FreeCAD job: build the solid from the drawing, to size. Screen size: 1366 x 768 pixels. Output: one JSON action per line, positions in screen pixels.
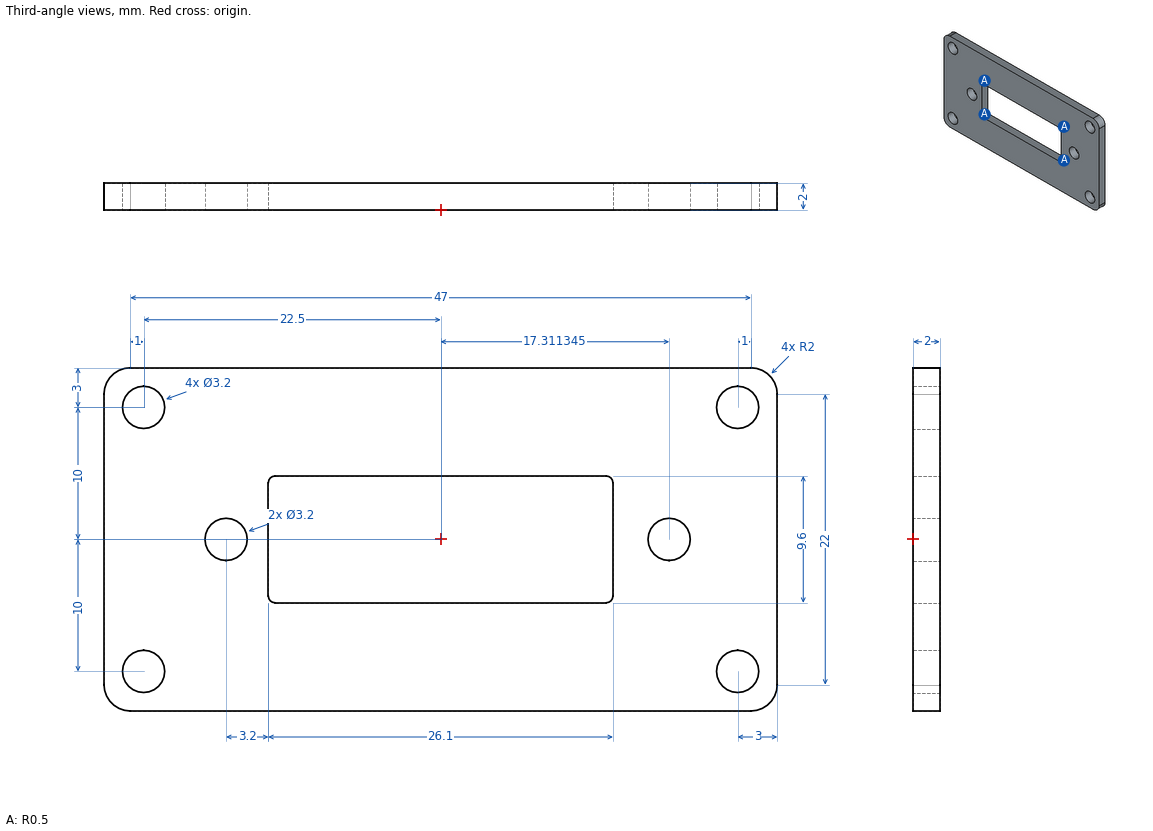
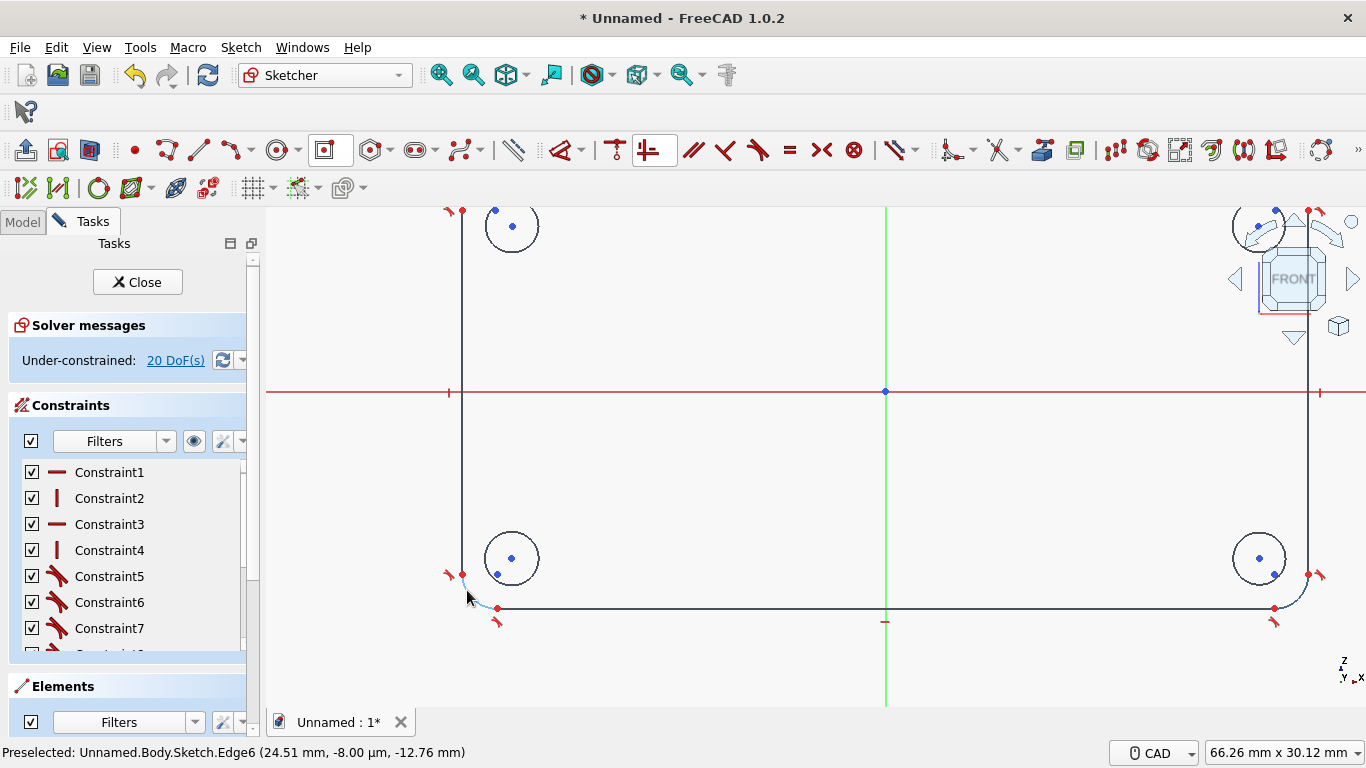
{"action": "left_click", "coordinate": [466, 590]}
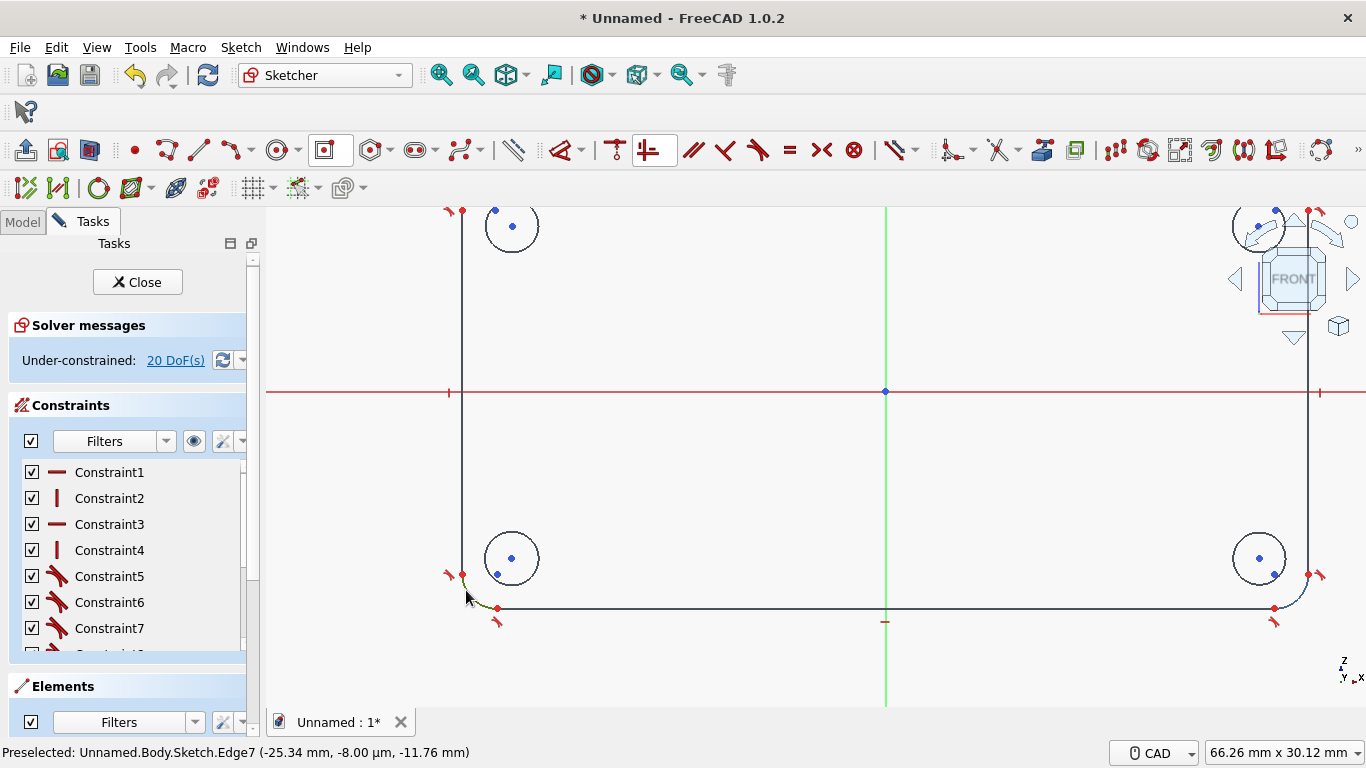
{"action": "scroll", "coordinate": [467, 590], "scroll_direction": "down", "scroll_amount": 2}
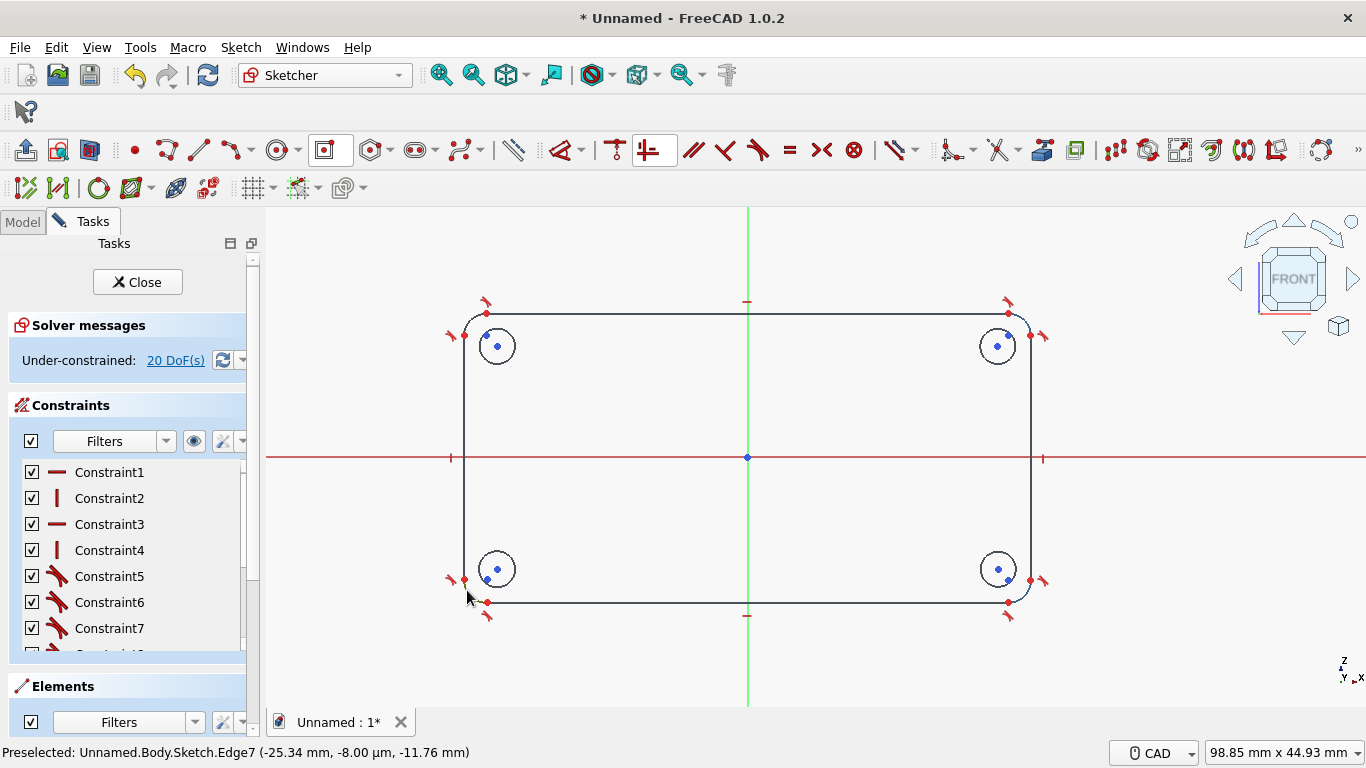
{"action": "scroll", "coordinate": [476, 316], "scroll_direction": "up", "scroll_amount": 2}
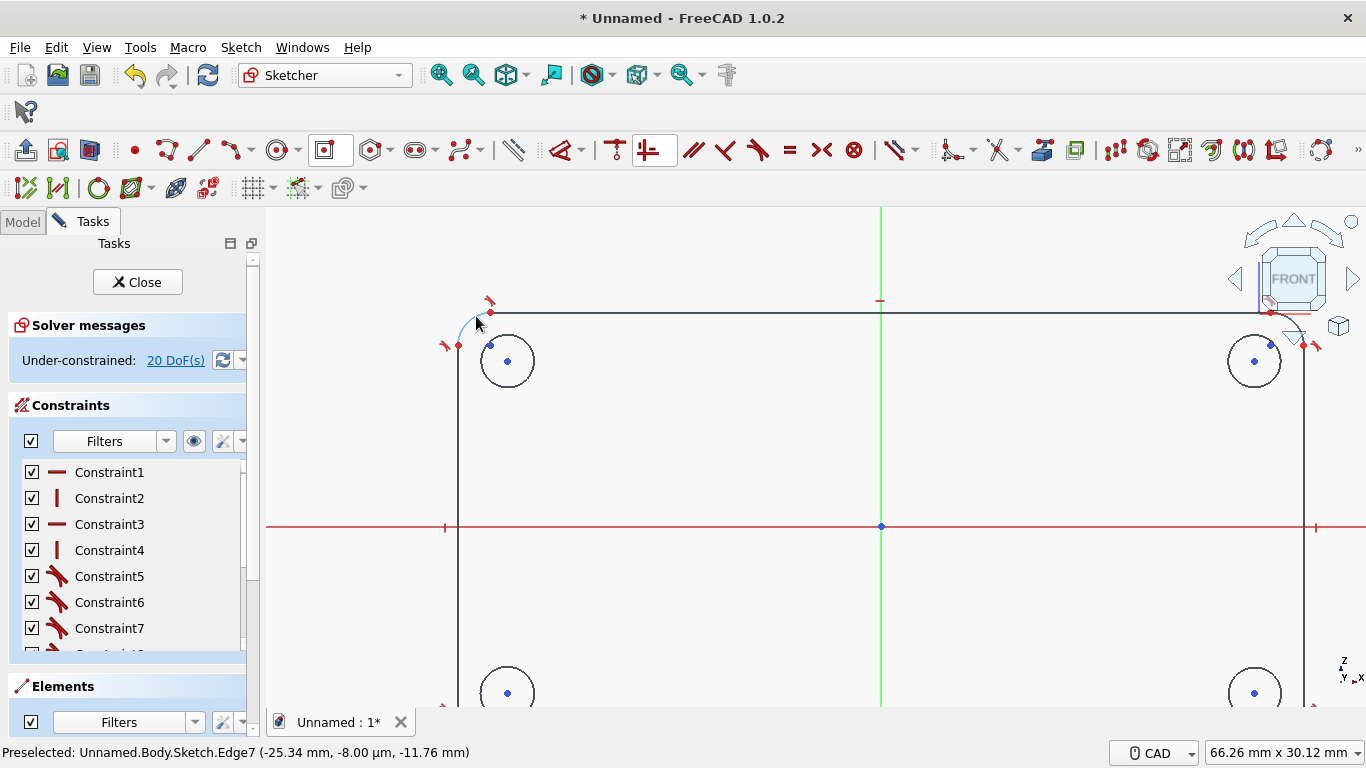
{"action": "left_click", "coordinate": [476, 316]}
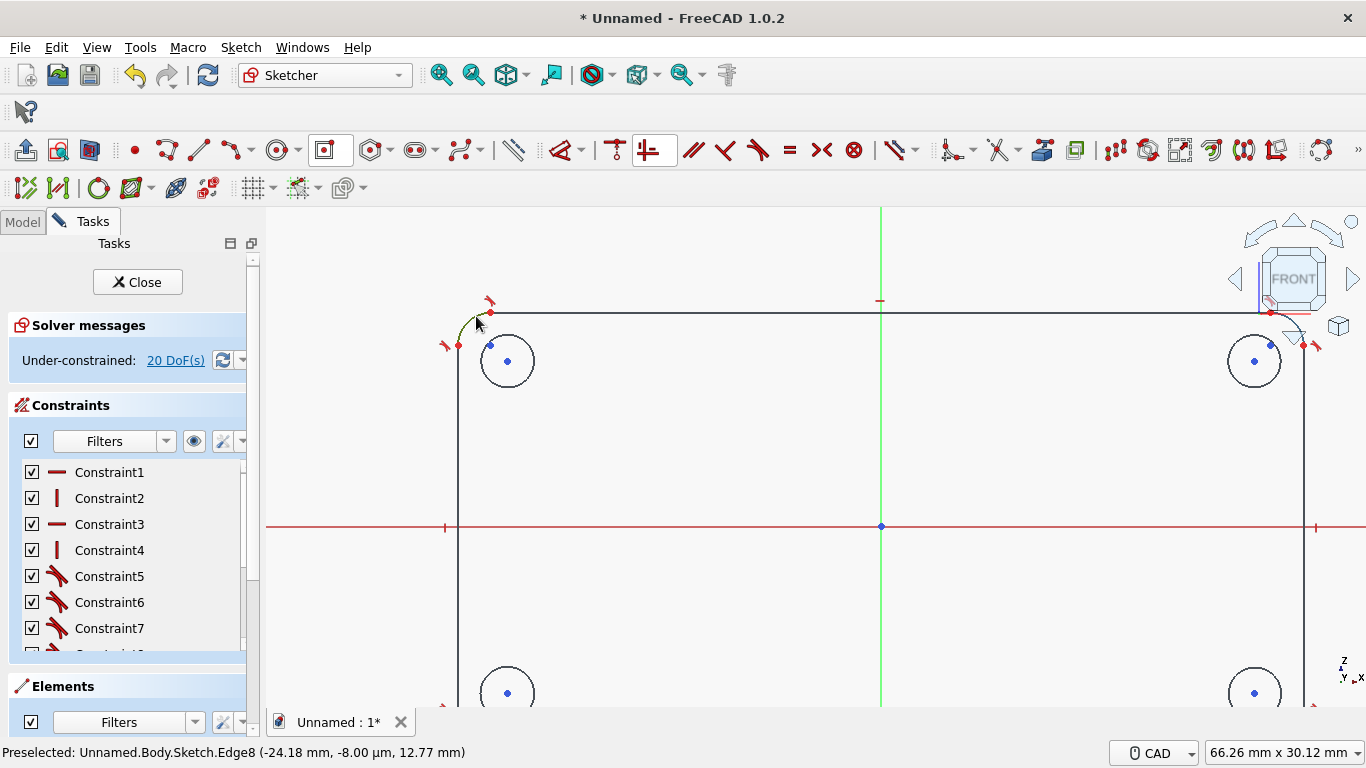
{"action": "left_click", "coordinate": [790, 150]}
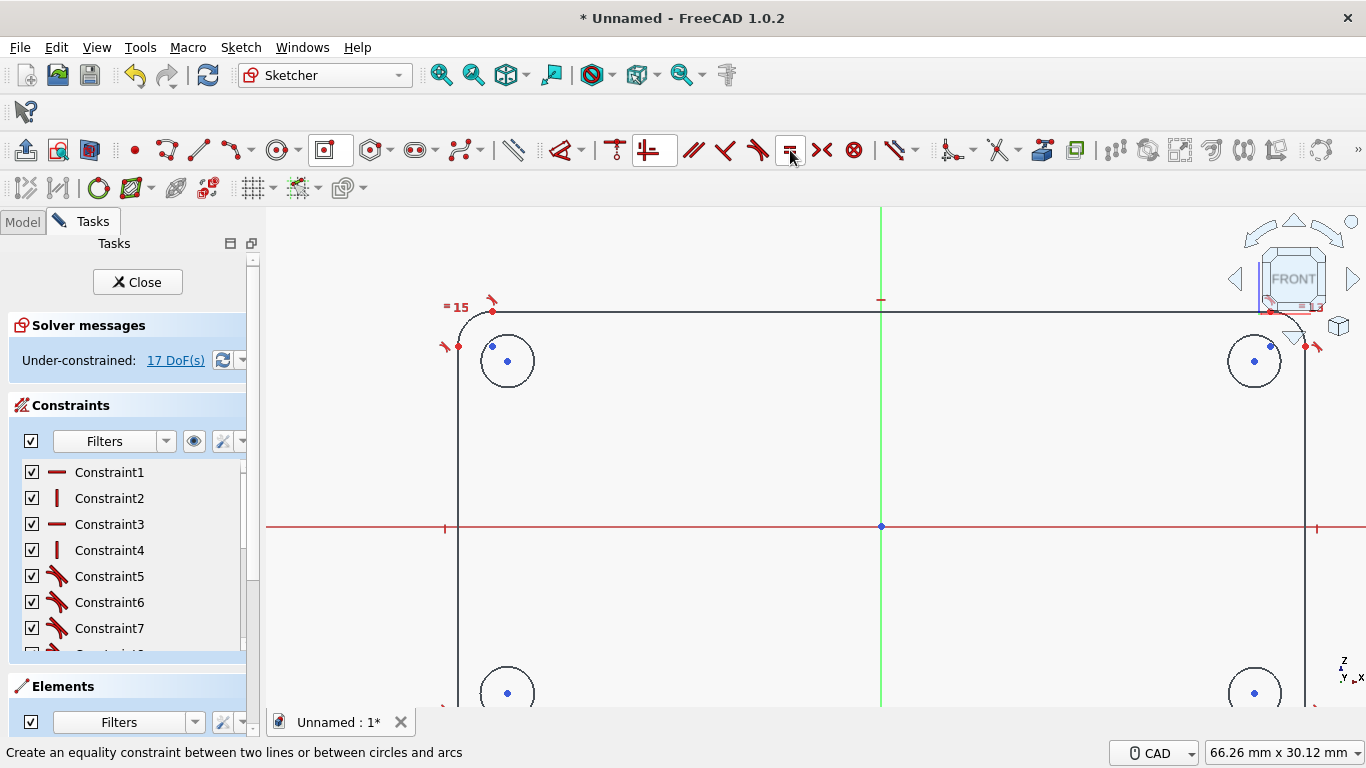
{"action": "left_click", "coordinate": [526, 342]}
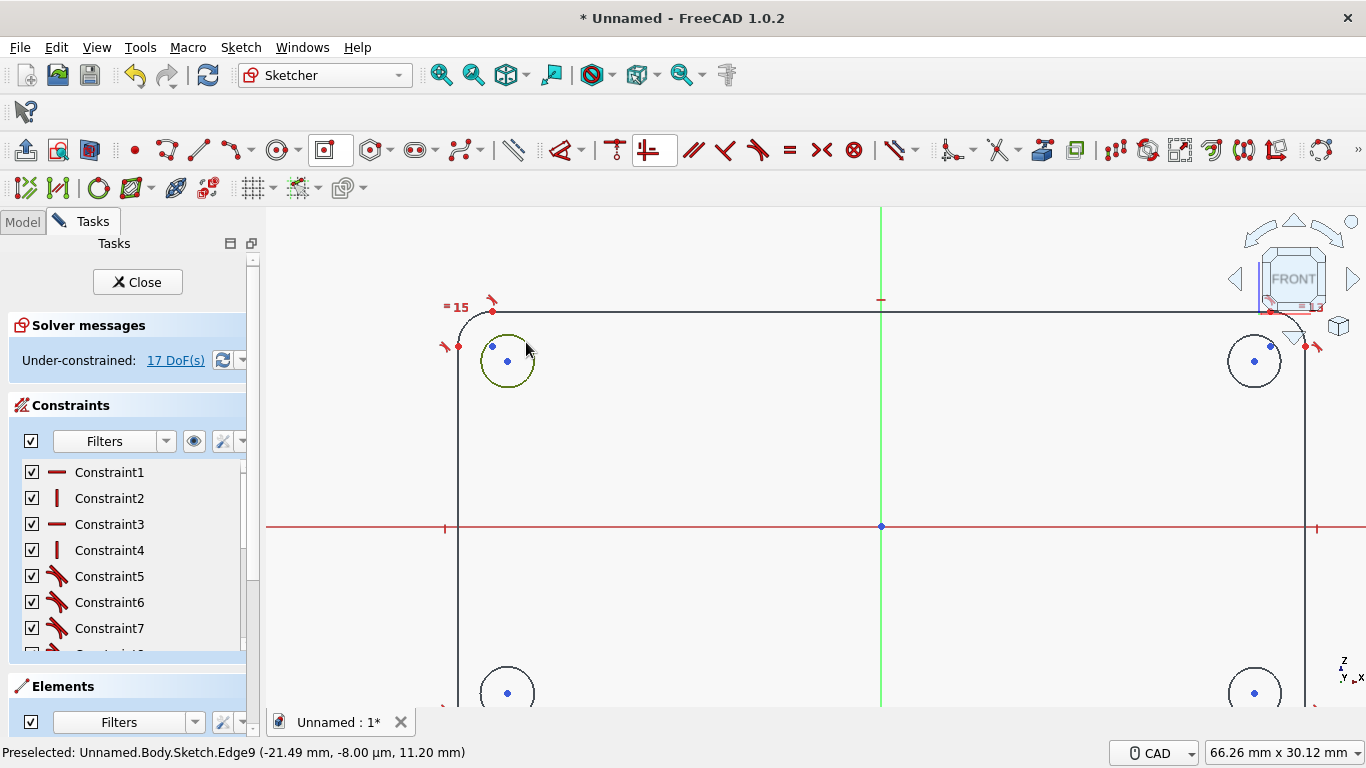
{"action": "scroll", "coordinate": [476, 315], "scroll_direction": "down", "scroll_amount": 2}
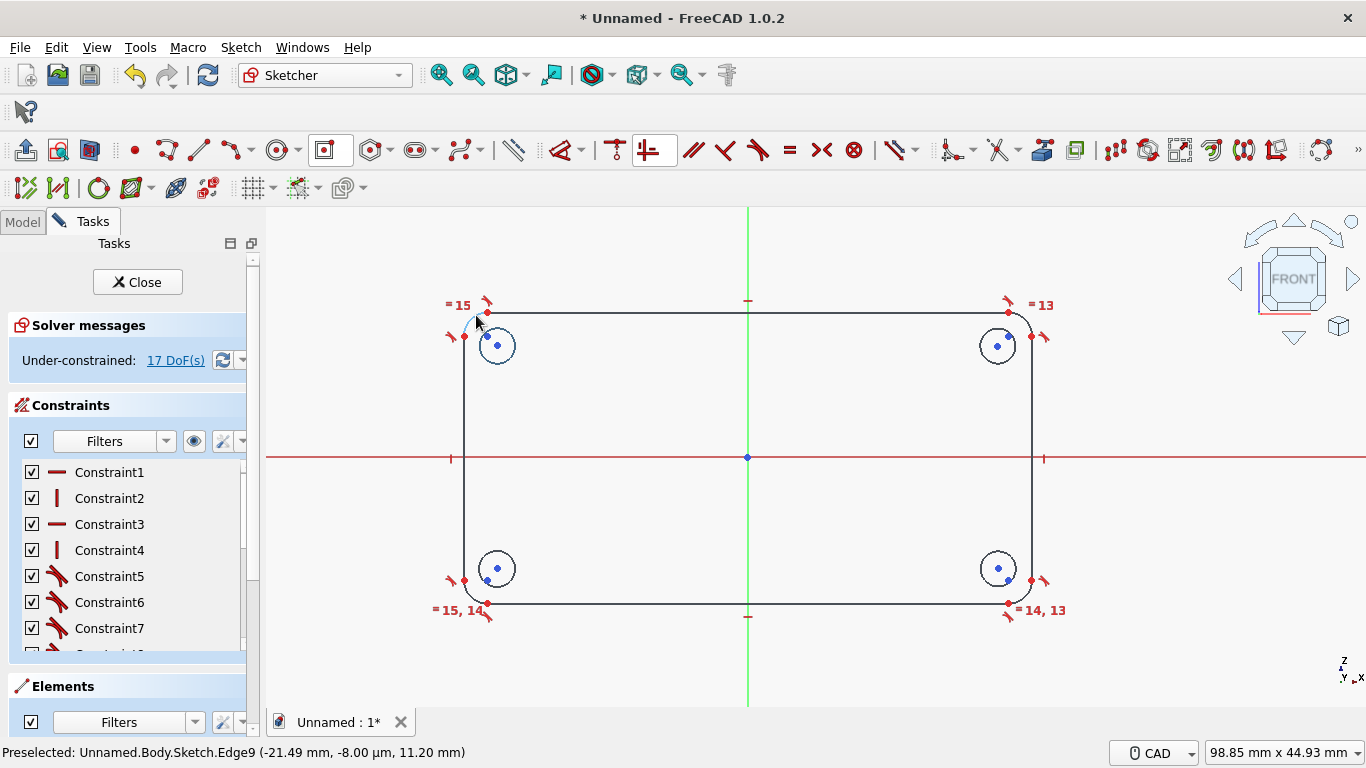
{"action": "left_click", "coordinate": [985, 334]}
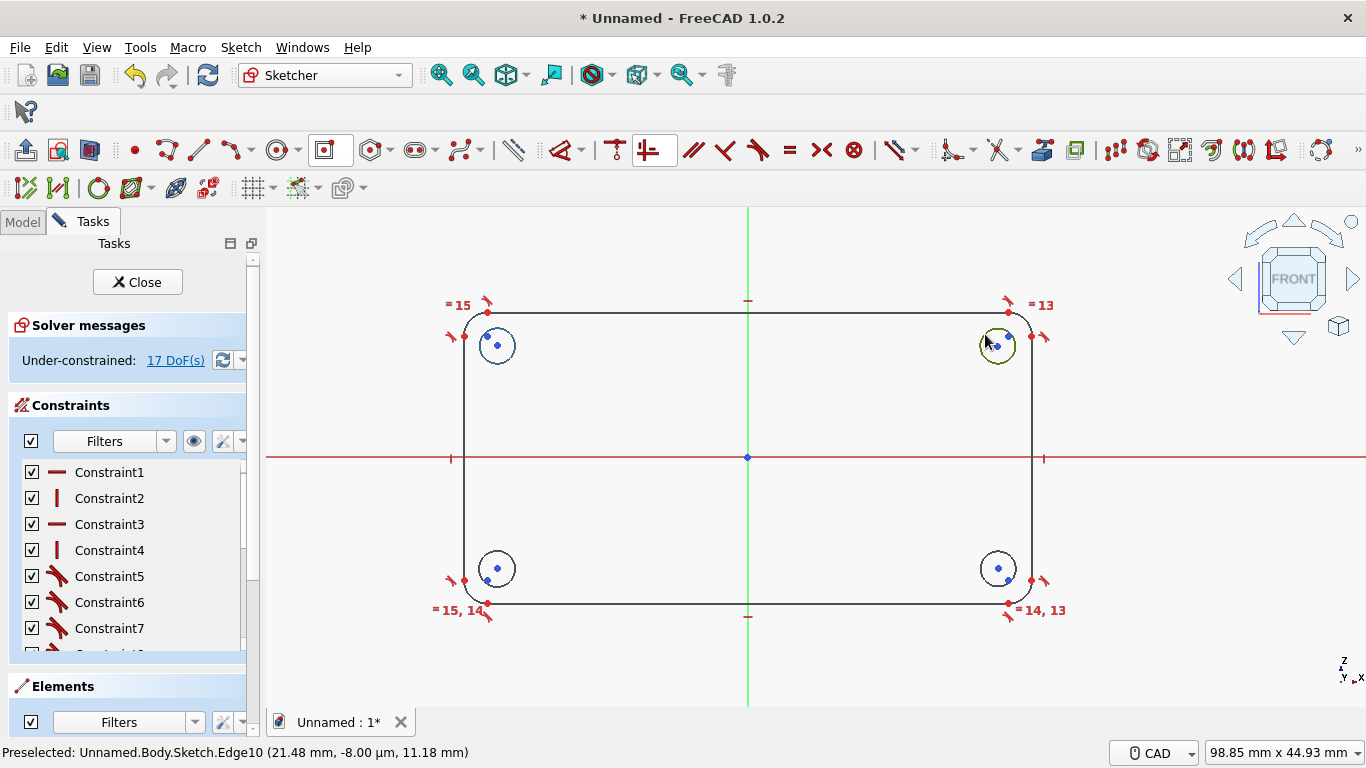
{"action": "left_click", "coordinate": [510, 556]}